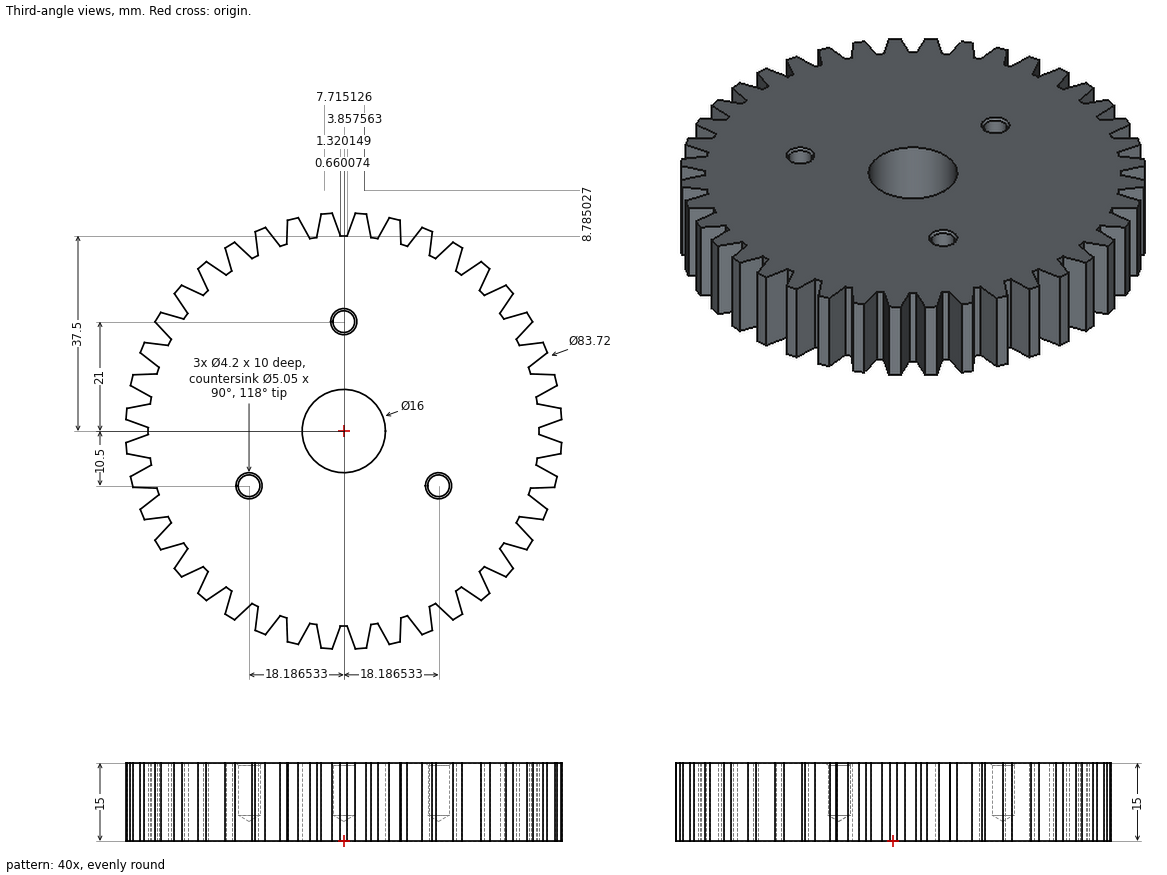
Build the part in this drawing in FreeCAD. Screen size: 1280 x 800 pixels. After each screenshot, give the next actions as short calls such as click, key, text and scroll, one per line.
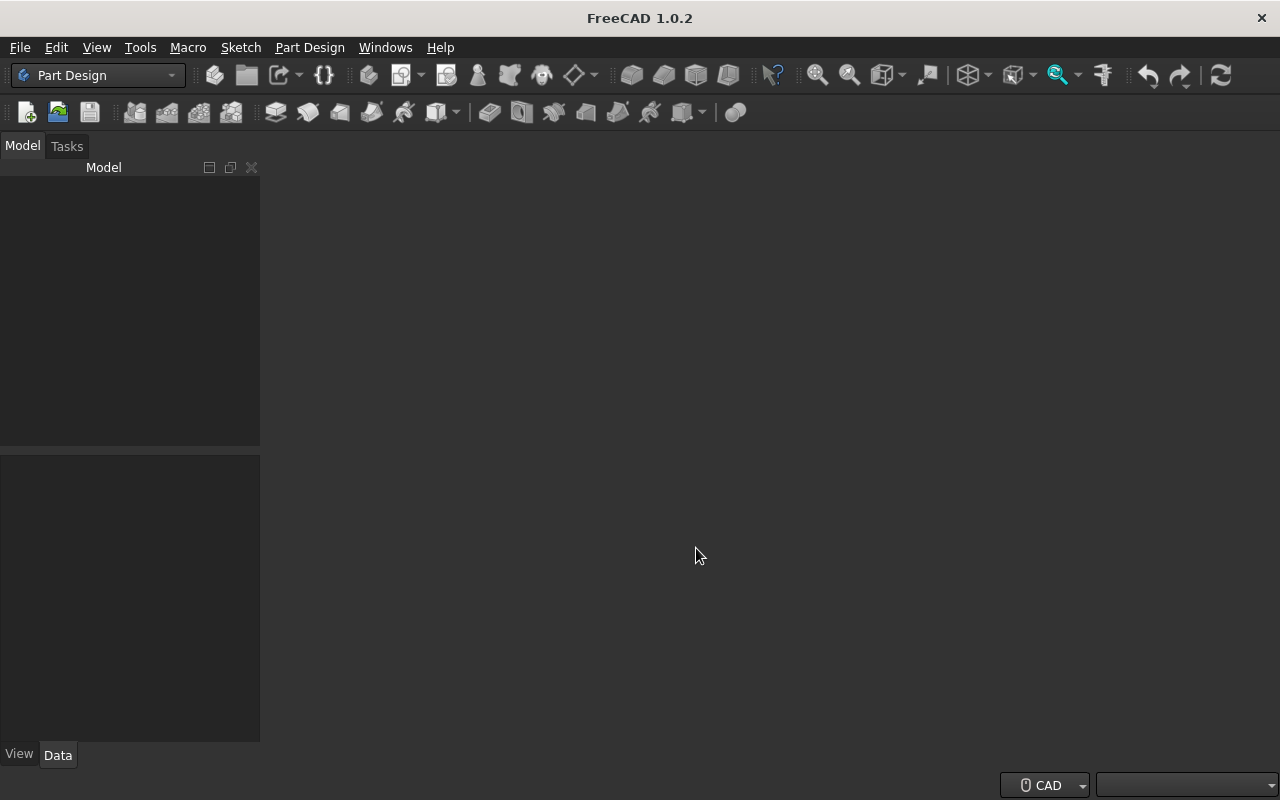
key(ctrl+n)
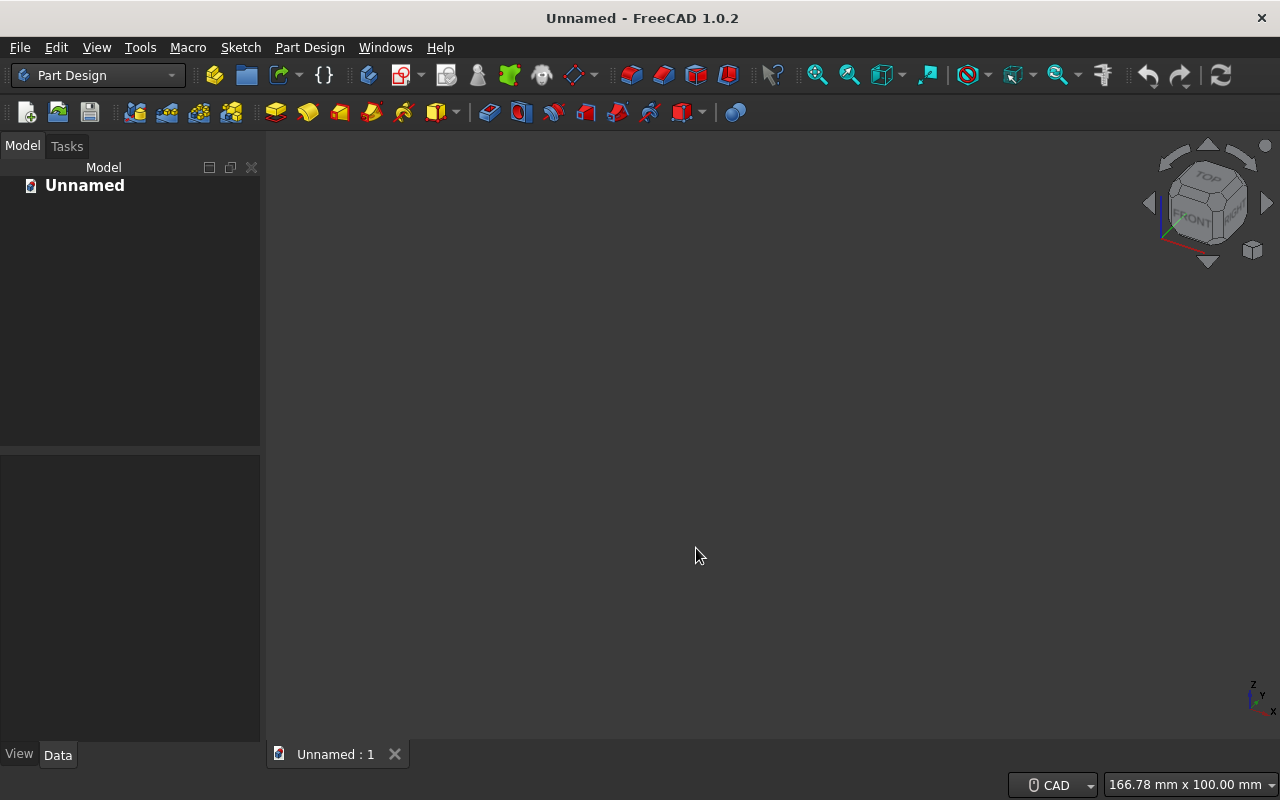
click(402, 76)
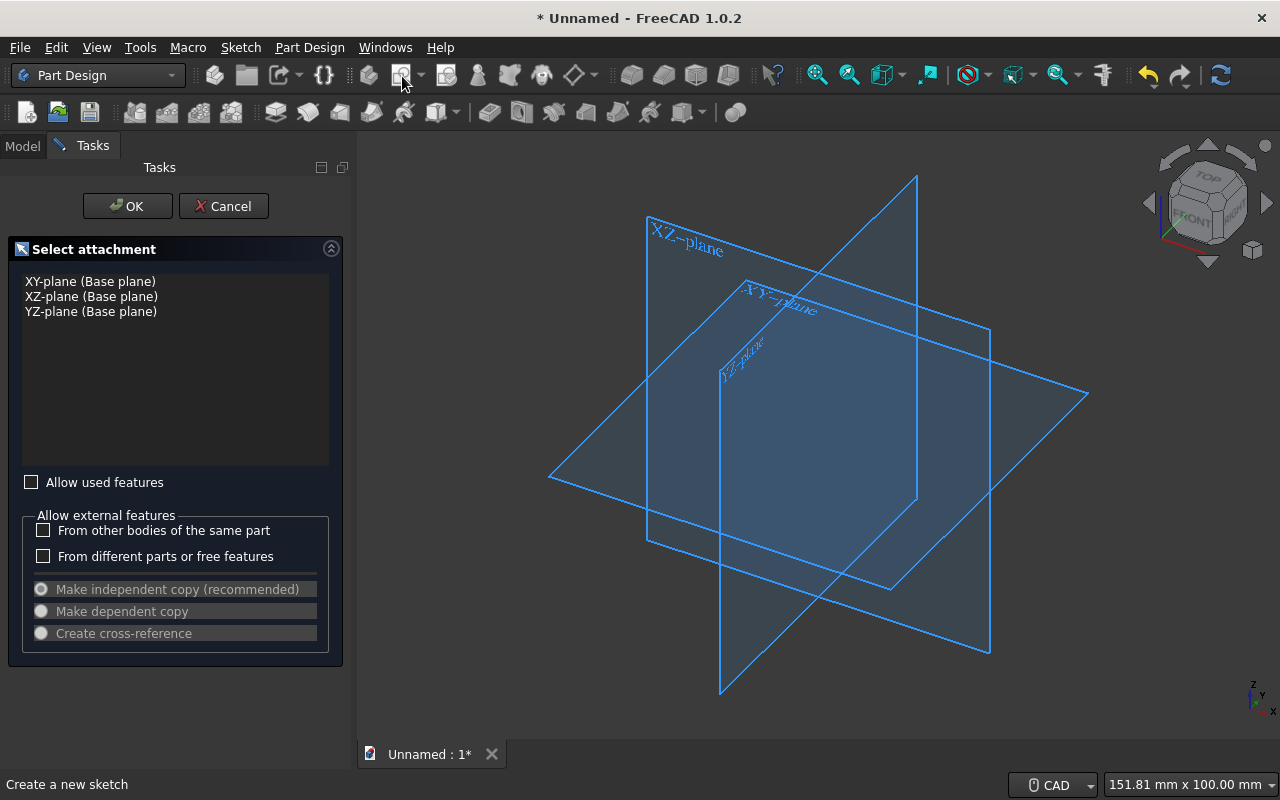
click(82, 282)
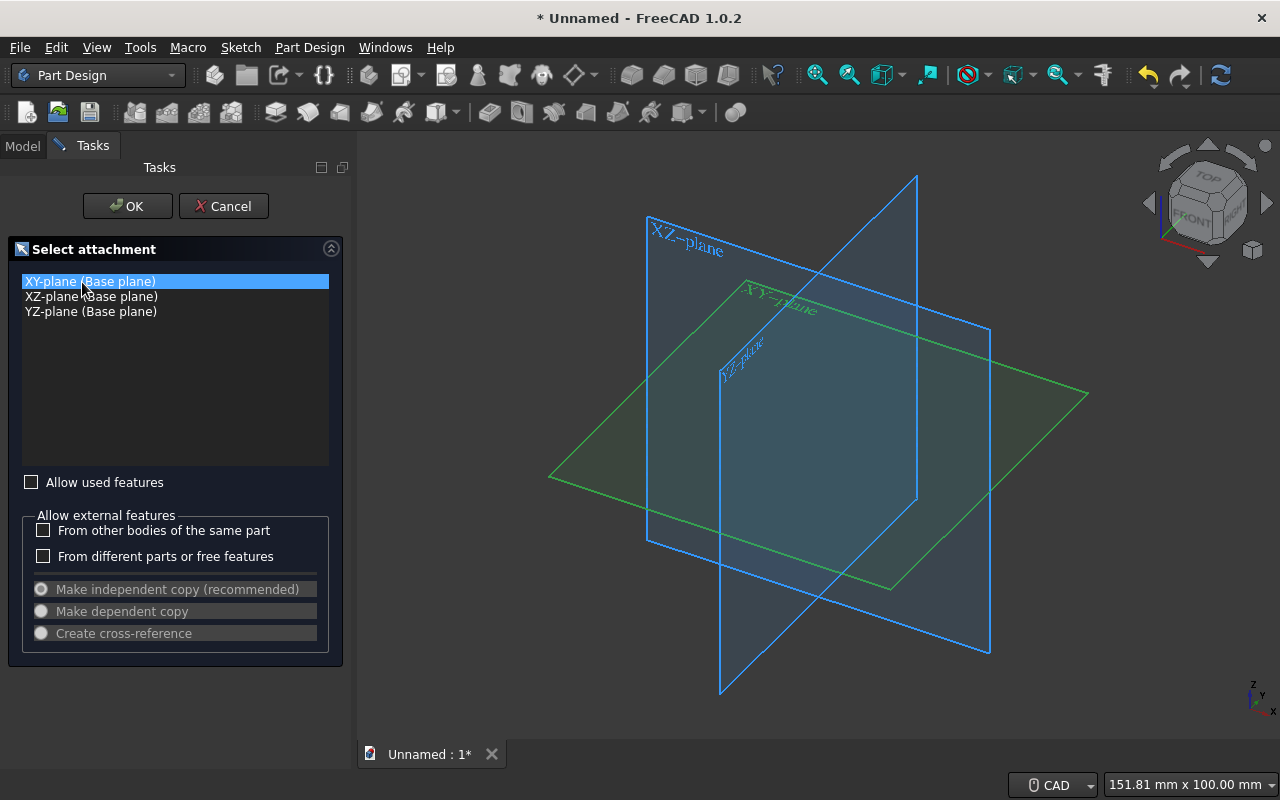
click(128, 206)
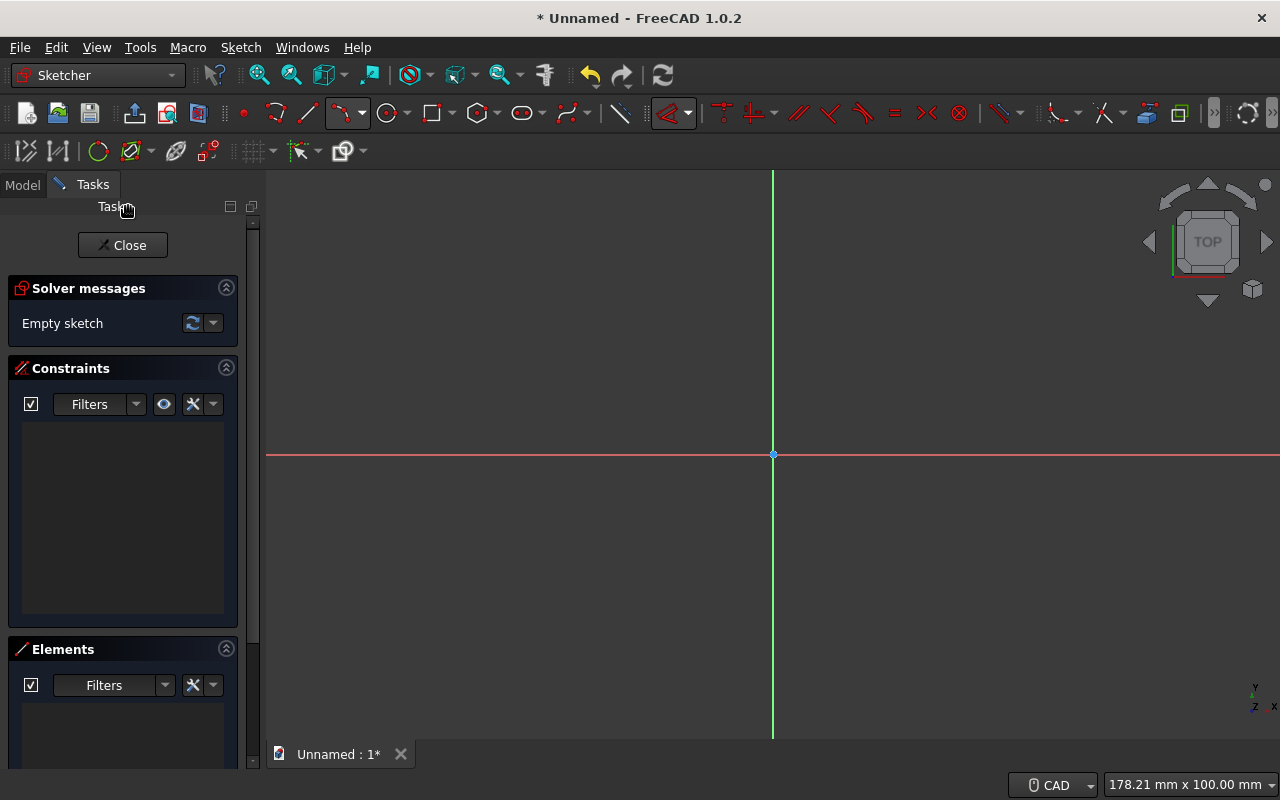
scroll(395, 455, down, 1)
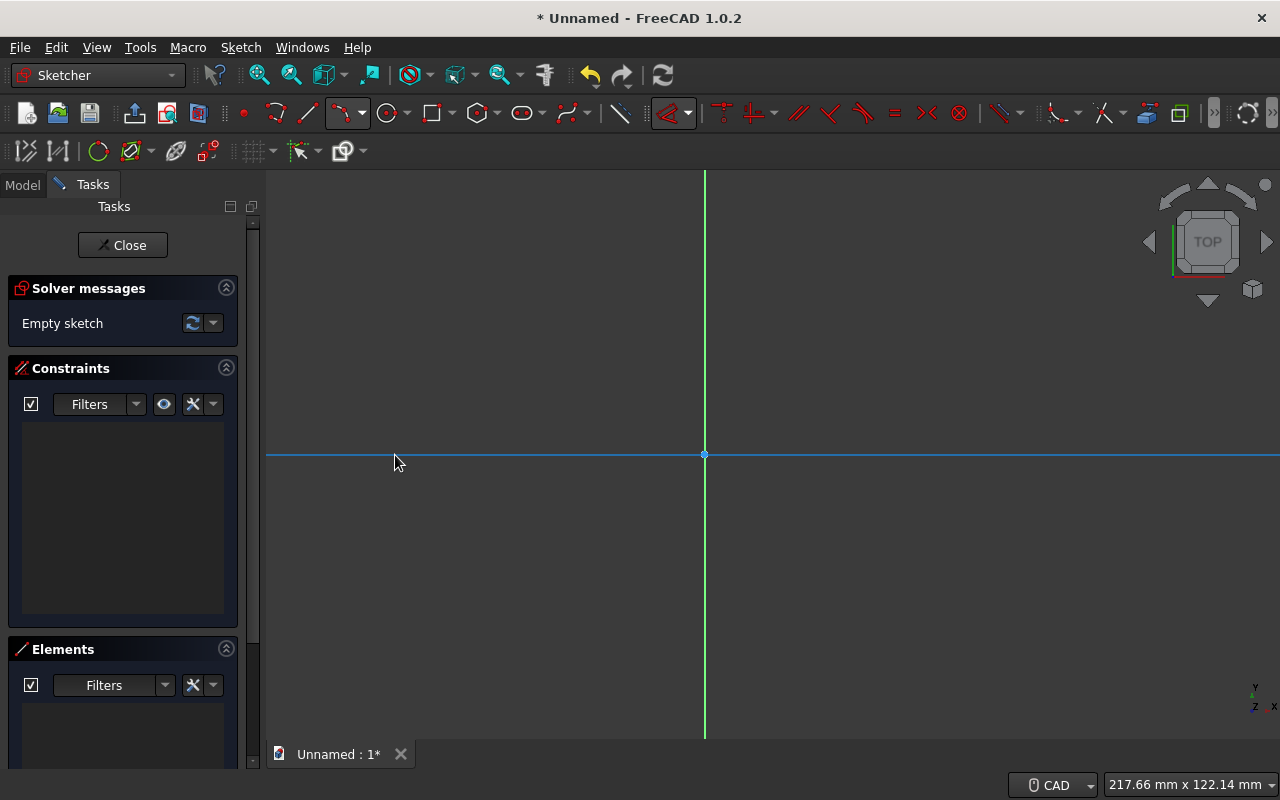
click(388, 114)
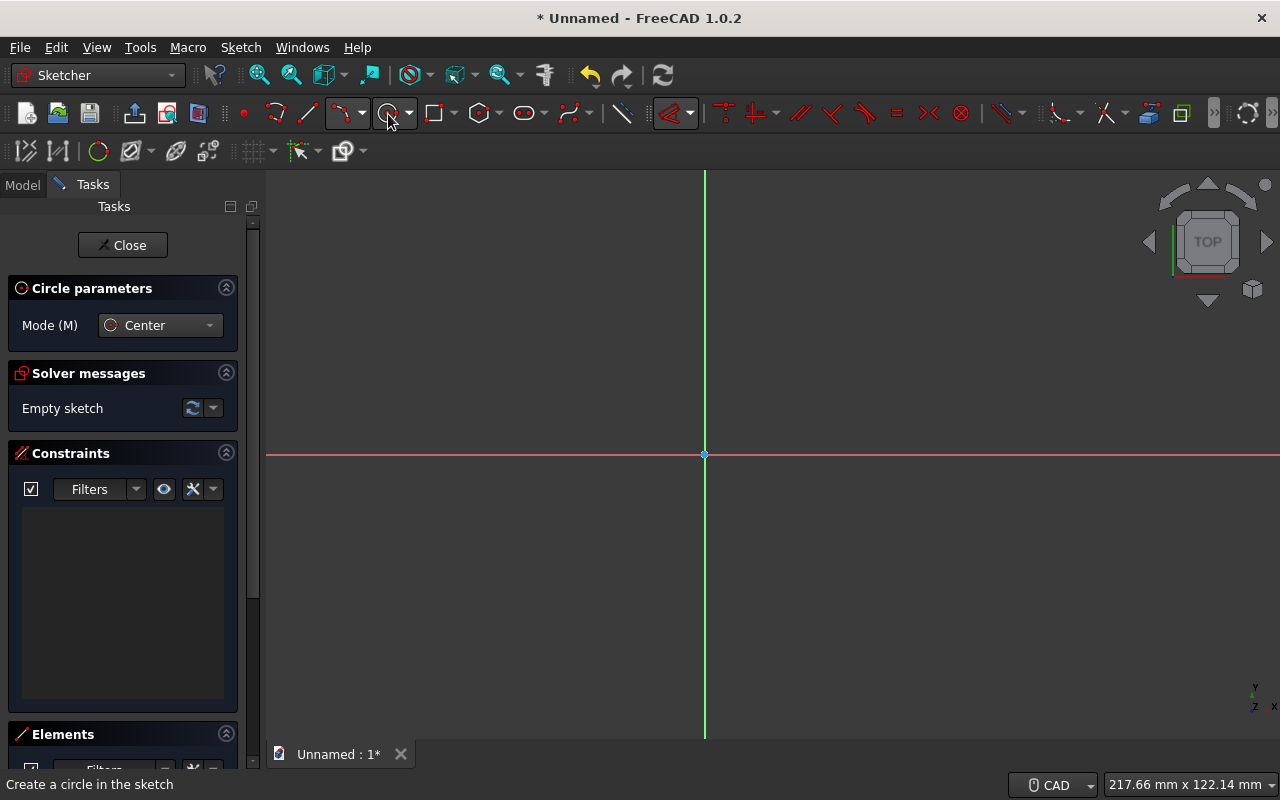
click(705, 455)
click(842, 317)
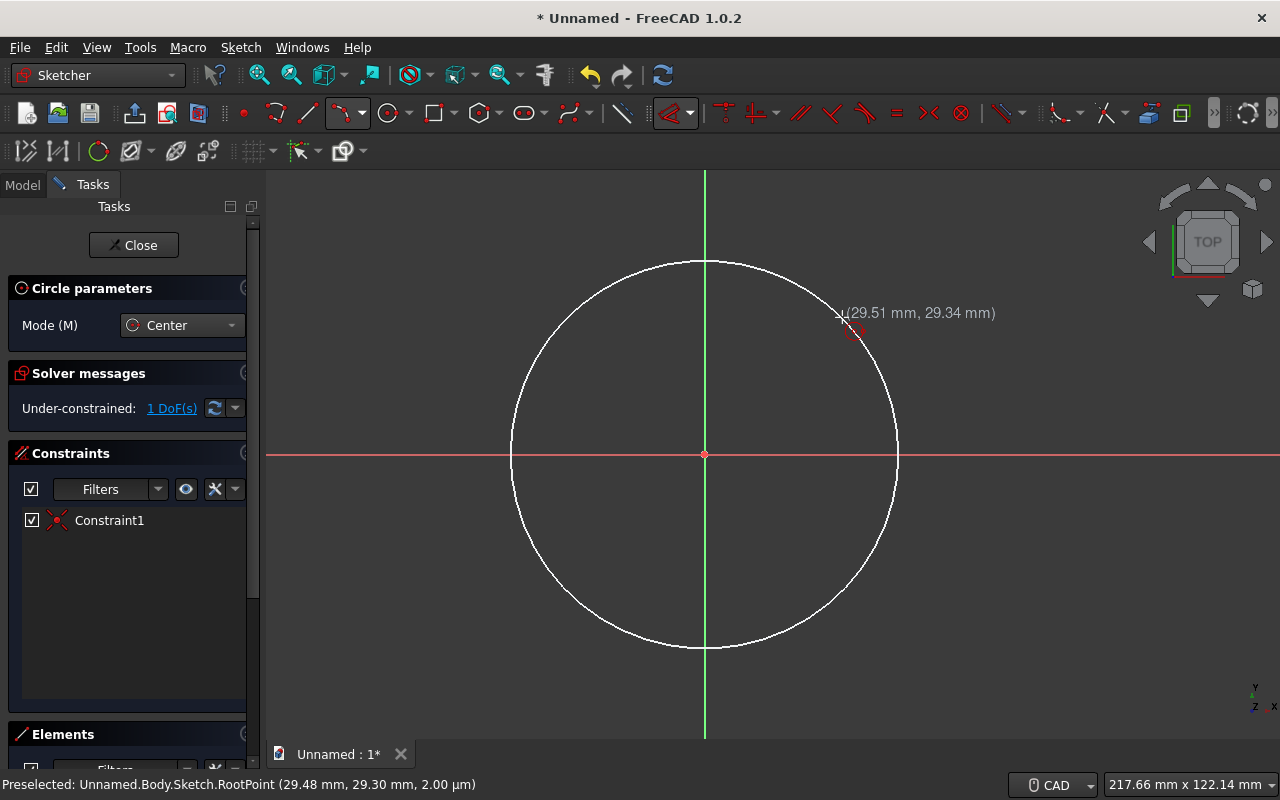
click(705, 455)
click(731, 428)
key(Escape)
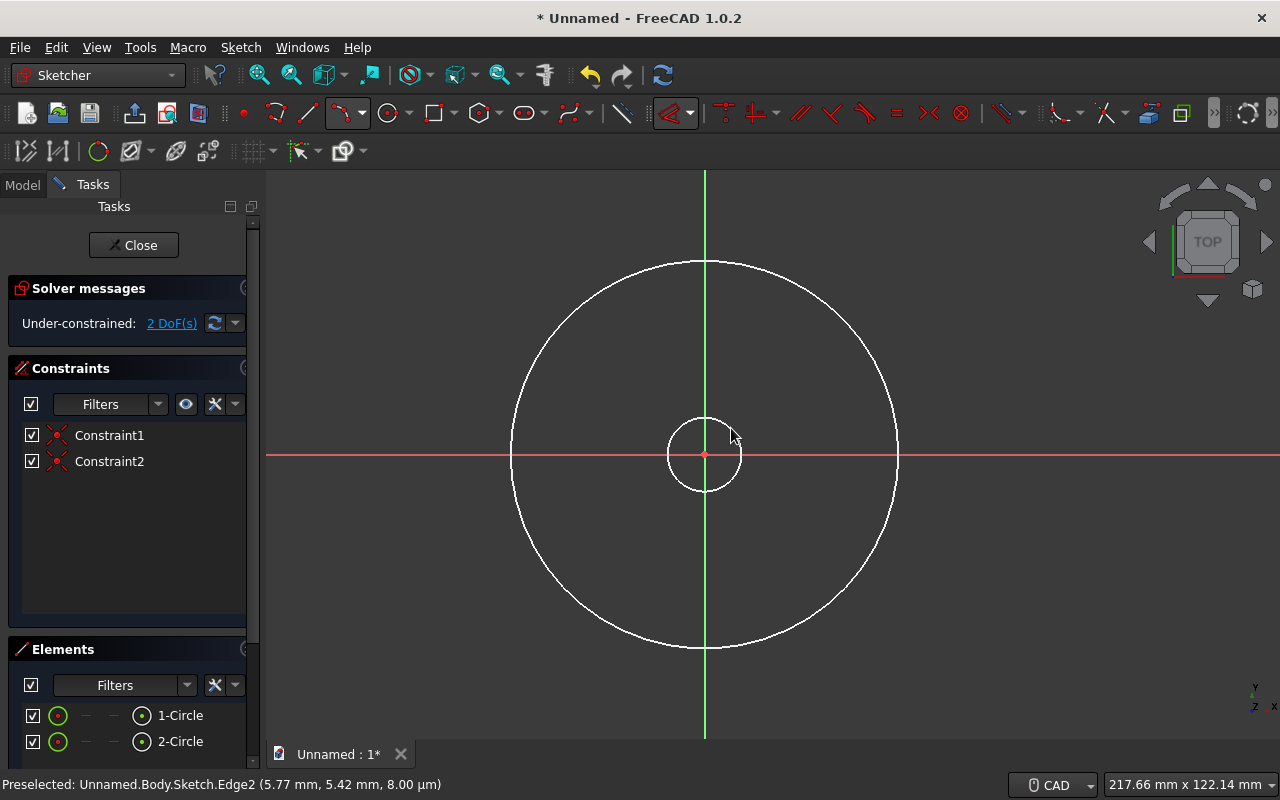
key(d)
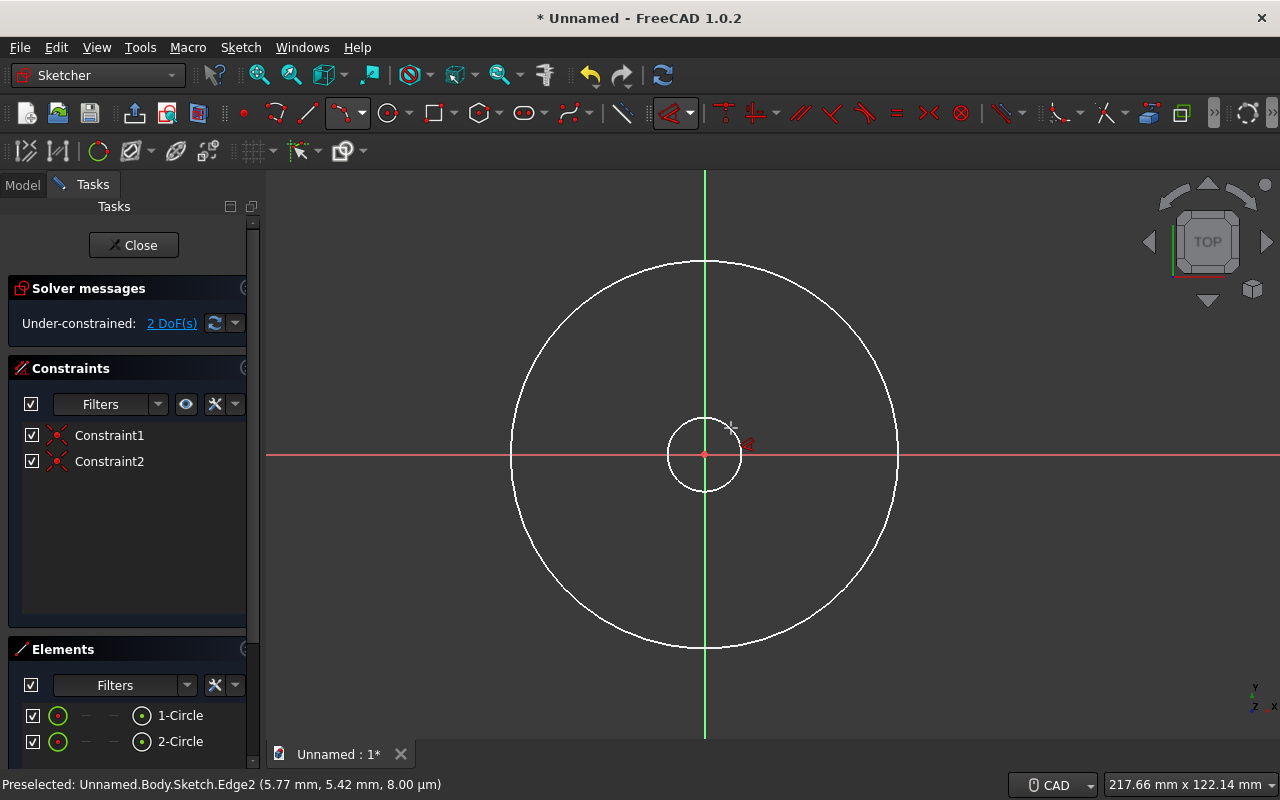
click(841, 317)
click(864, 294)